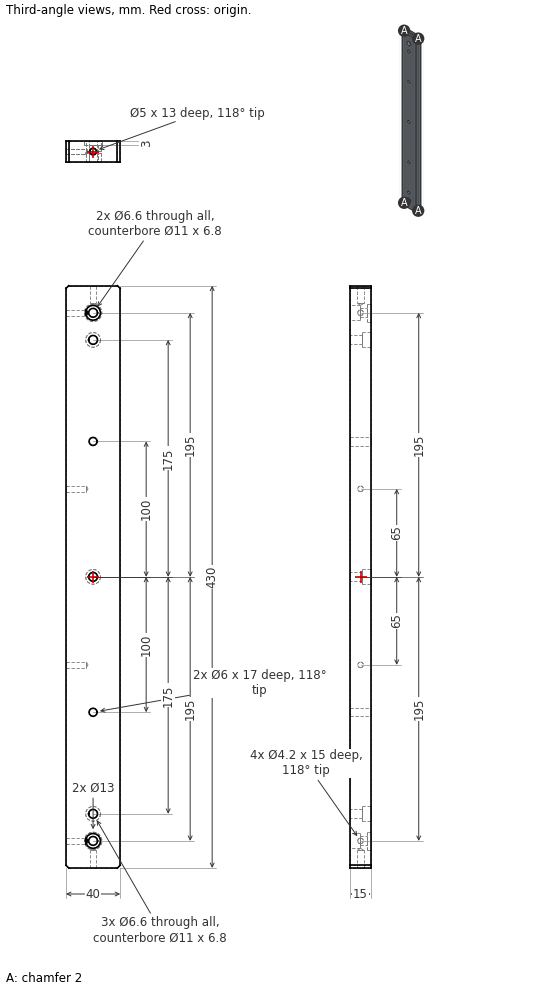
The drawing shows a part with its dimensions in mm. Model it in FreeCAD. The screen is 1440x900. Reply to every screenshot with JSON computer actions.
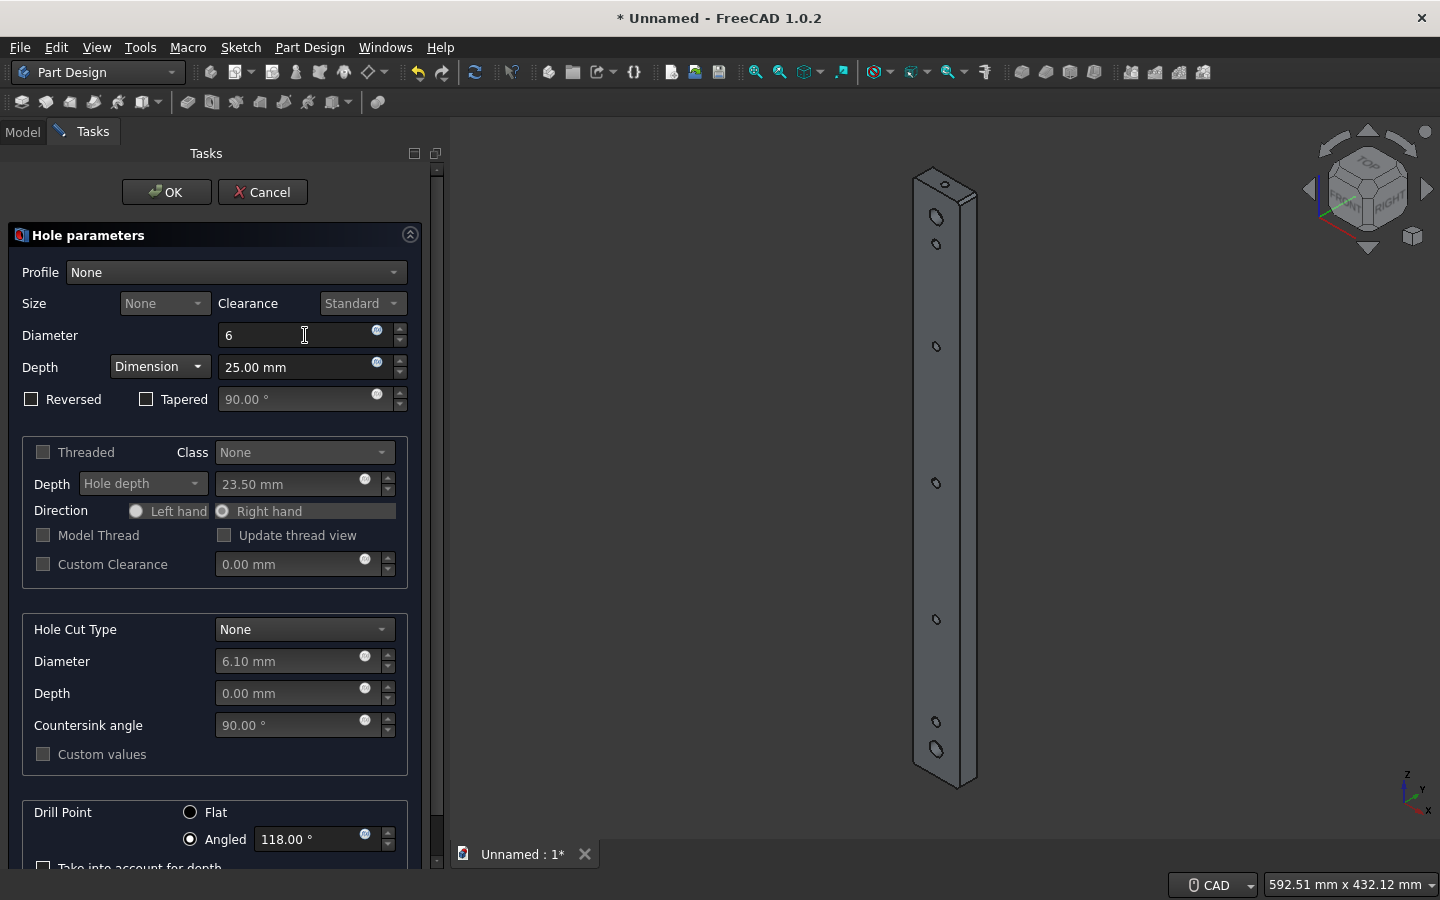
{"action": "triple_click", "coordinate": [305, 367]}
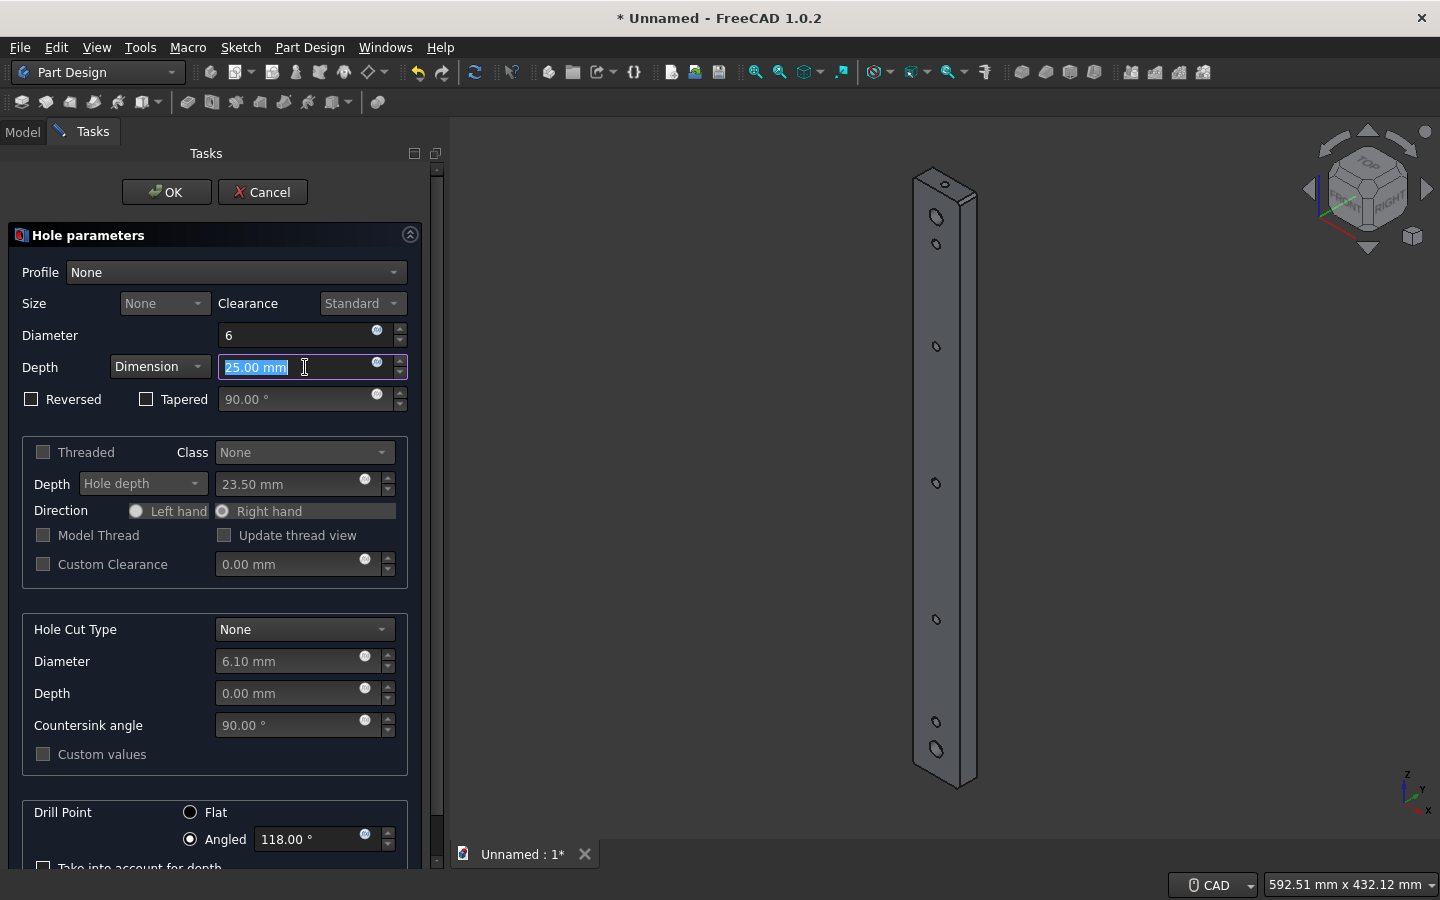
{"action": "type", "text": "17"}
{"action": "key", "text": "Tab"}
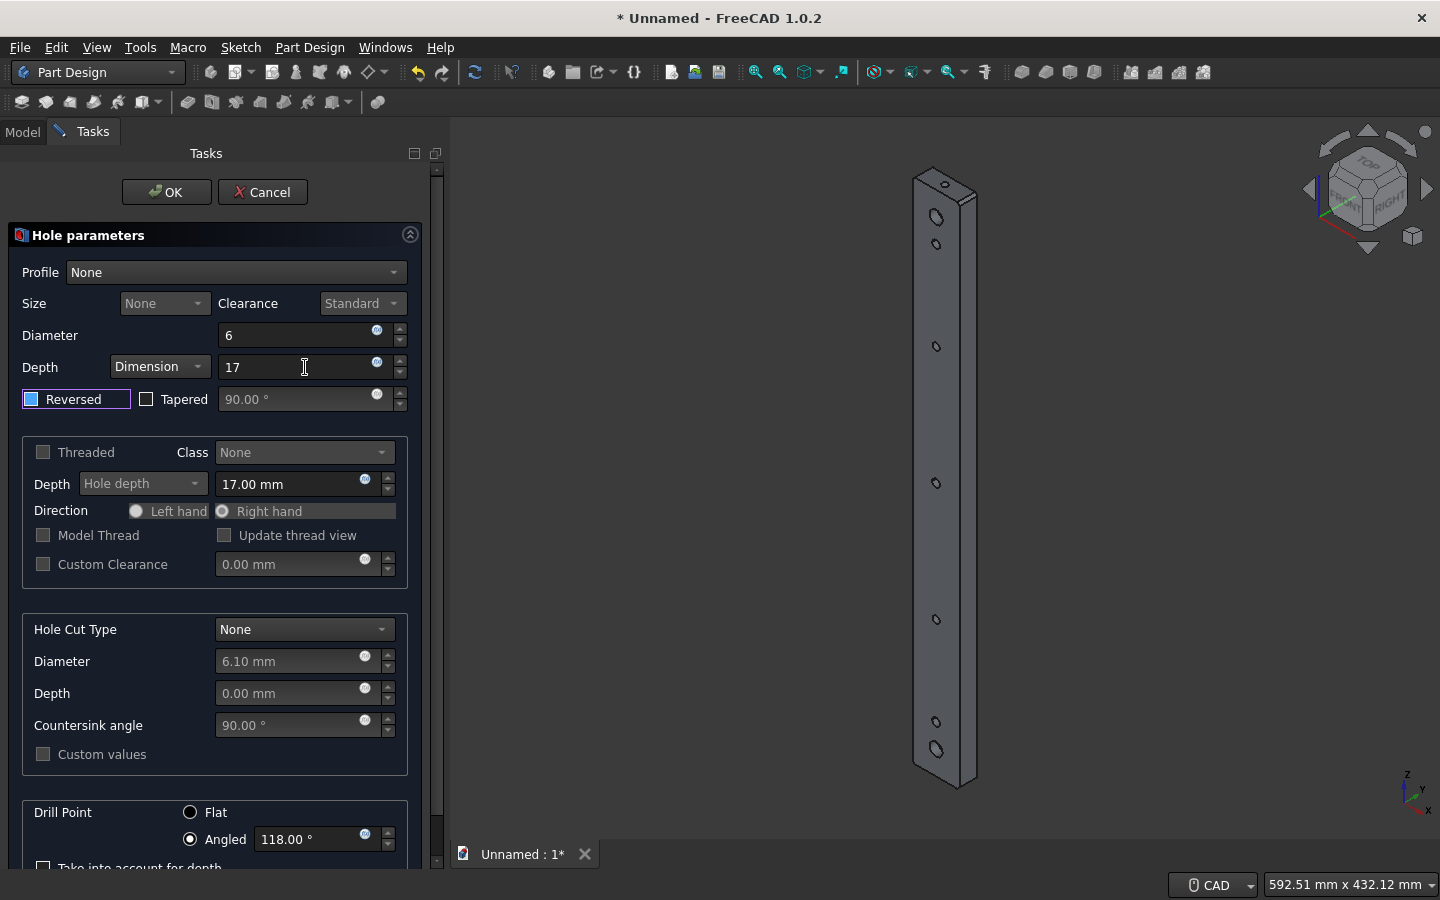
{"action": "left_click", "coordinate": [167, 192]}